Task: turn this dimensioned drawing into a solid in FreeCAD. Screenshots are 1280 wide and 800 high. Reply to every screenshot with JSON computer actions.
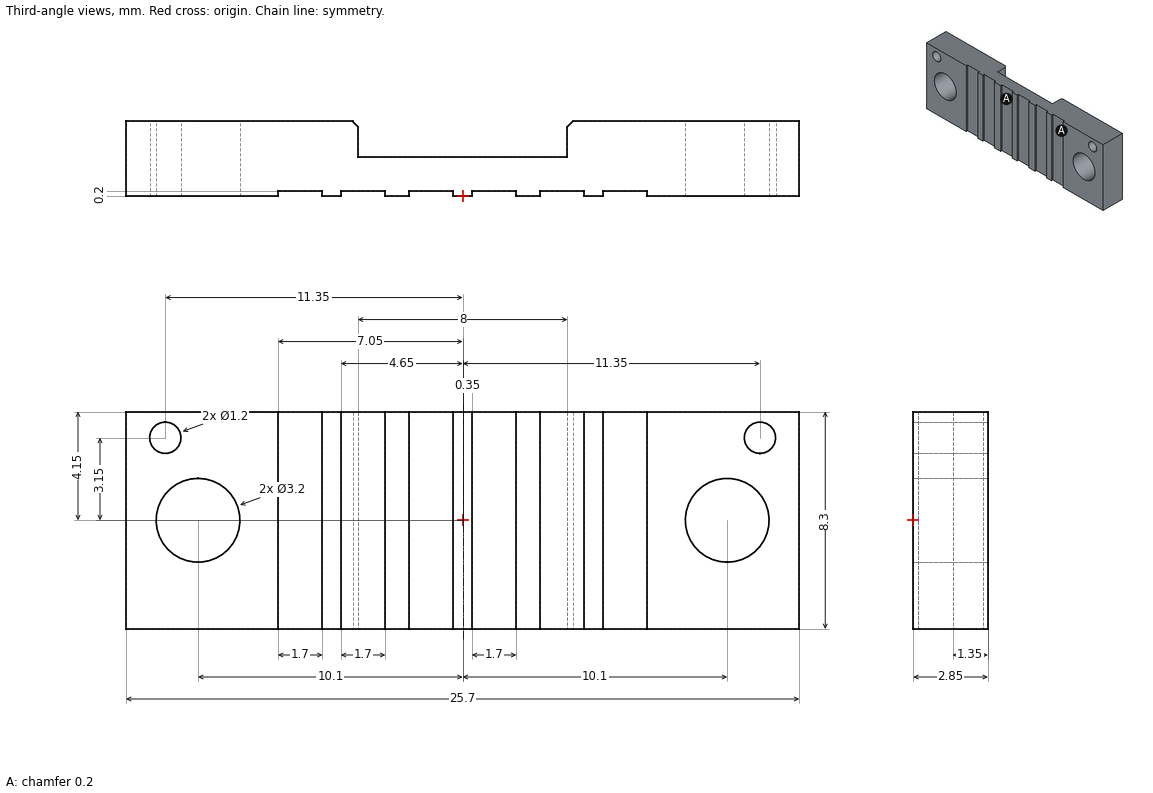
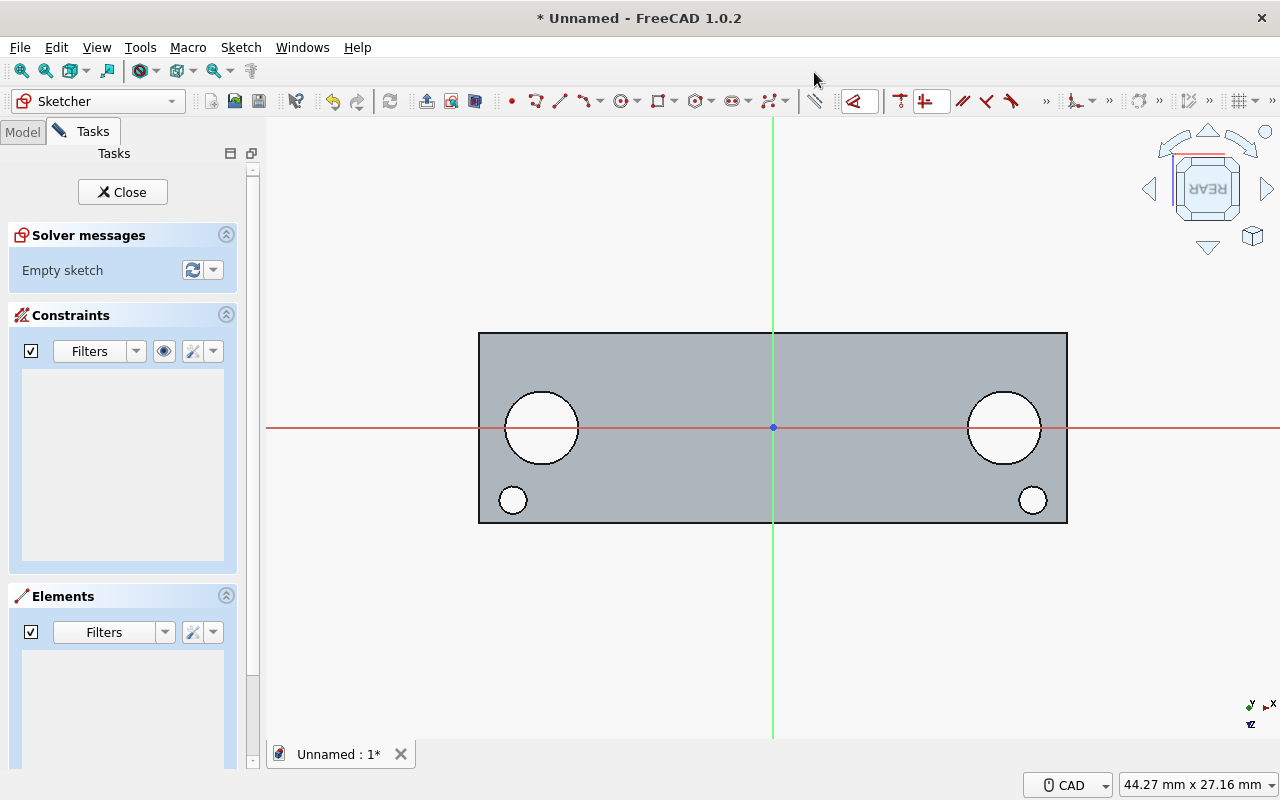
{"action": "scroll", "coordinate": [829, 428], "scroll_direction": "up", "scroll_amount": 4}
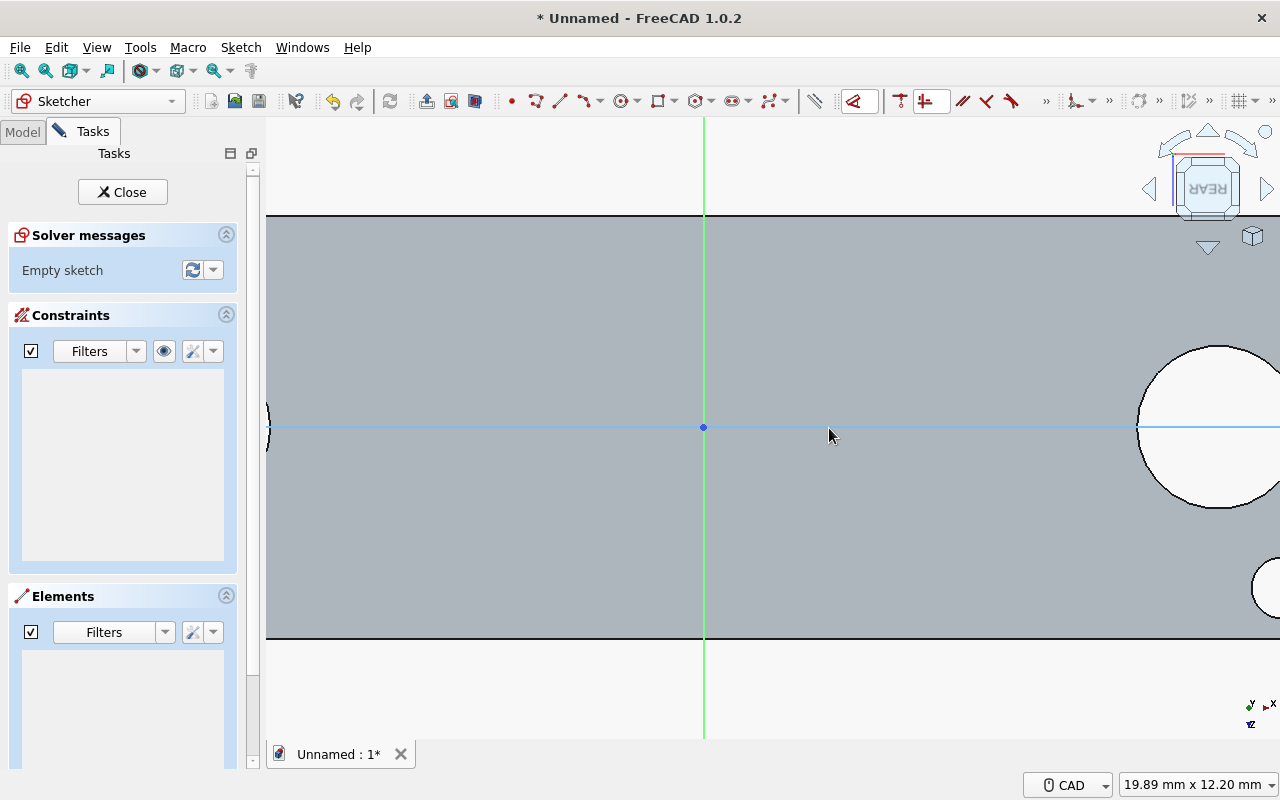
{"action": "key", "text": "g v"}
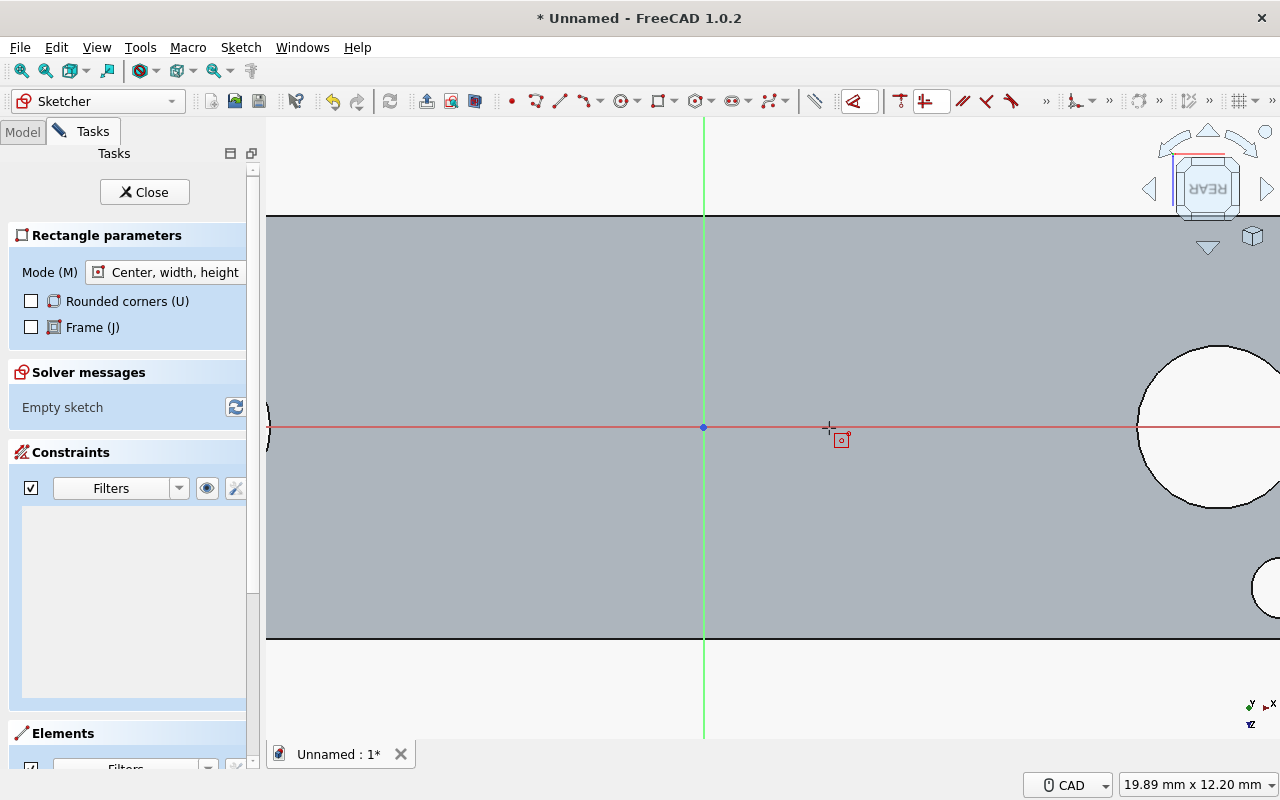
{"action": "left_click", "coordinate": [704, 427]}
{"action": "left_click", "coordinate": [908, 216]}
{"action": "key", "text": "Escape"}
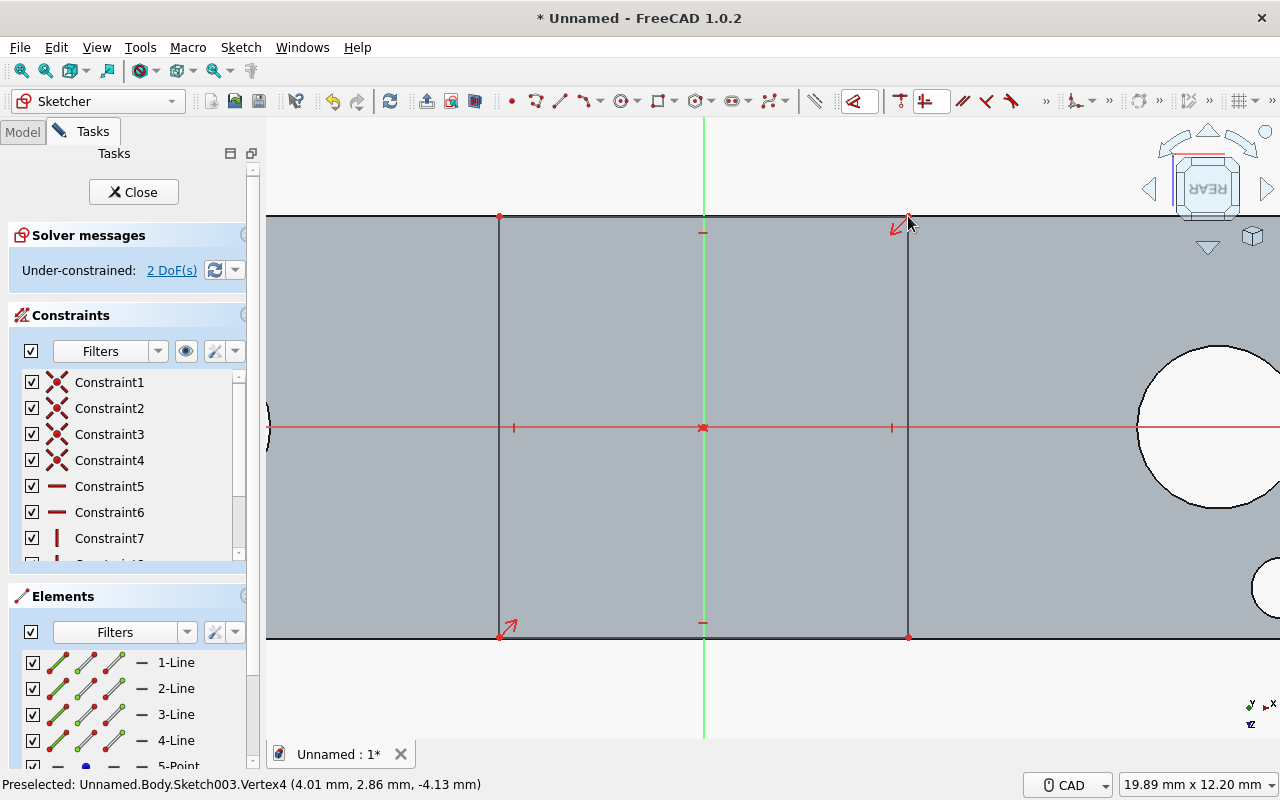
{"action": "key", "text": "d"}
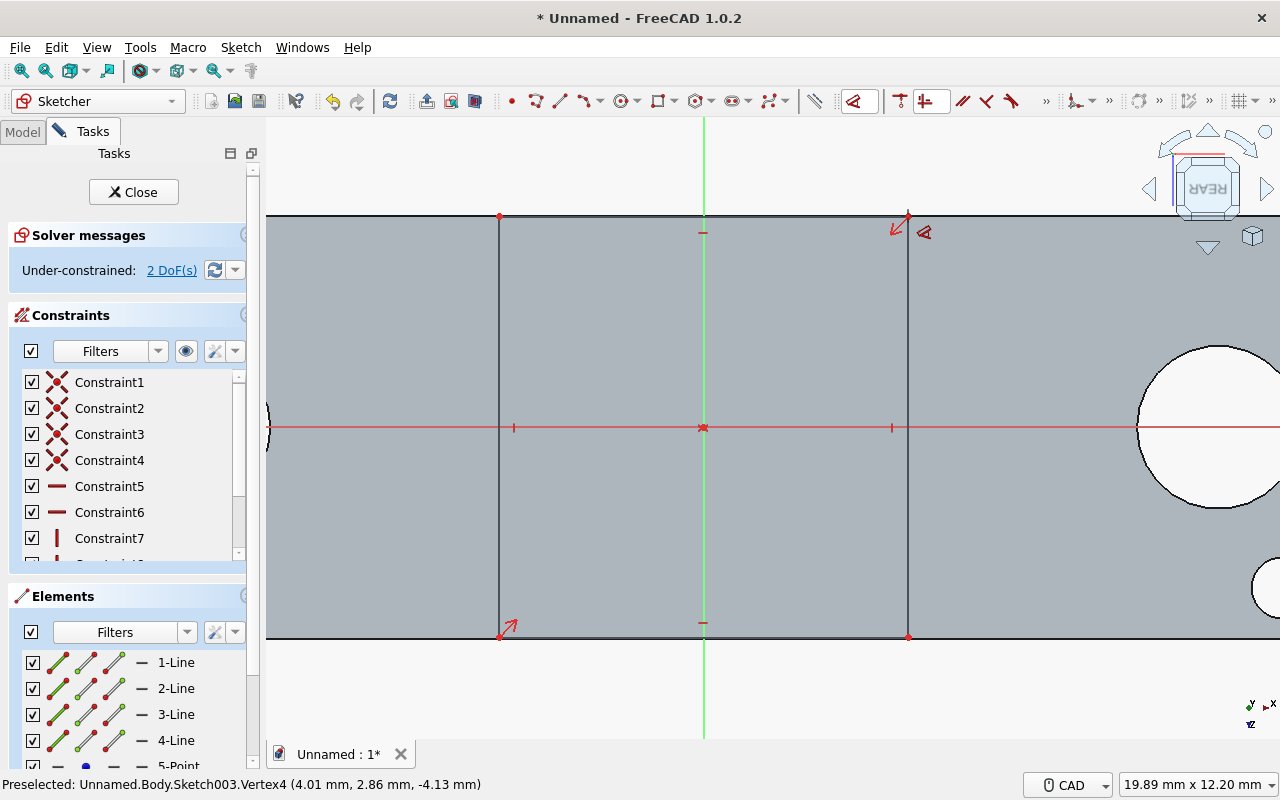
{"action": "left_click", "coordinate": [622, 638]}
{"action": "left_click", "coordinate": [610, 672]}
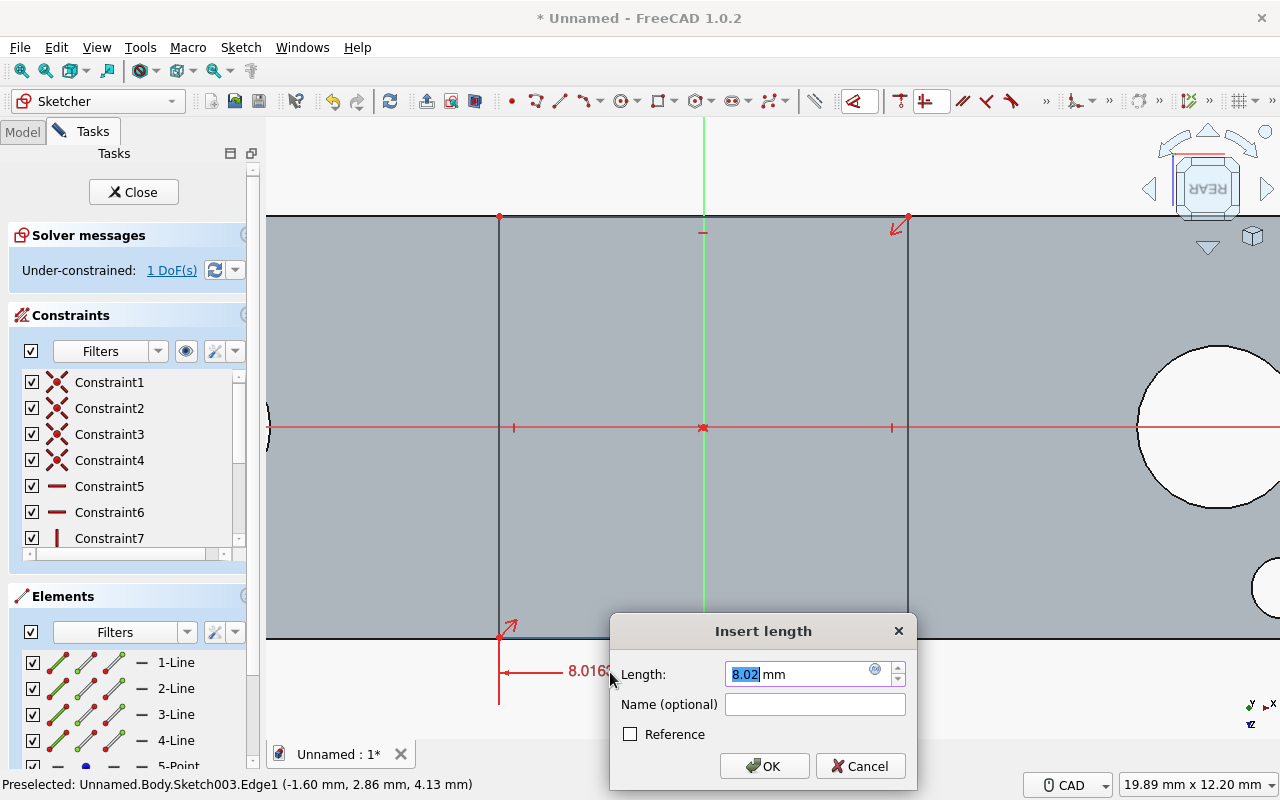
{"action": "type", "text": "8"}
{"action": "key", "text": "Return"}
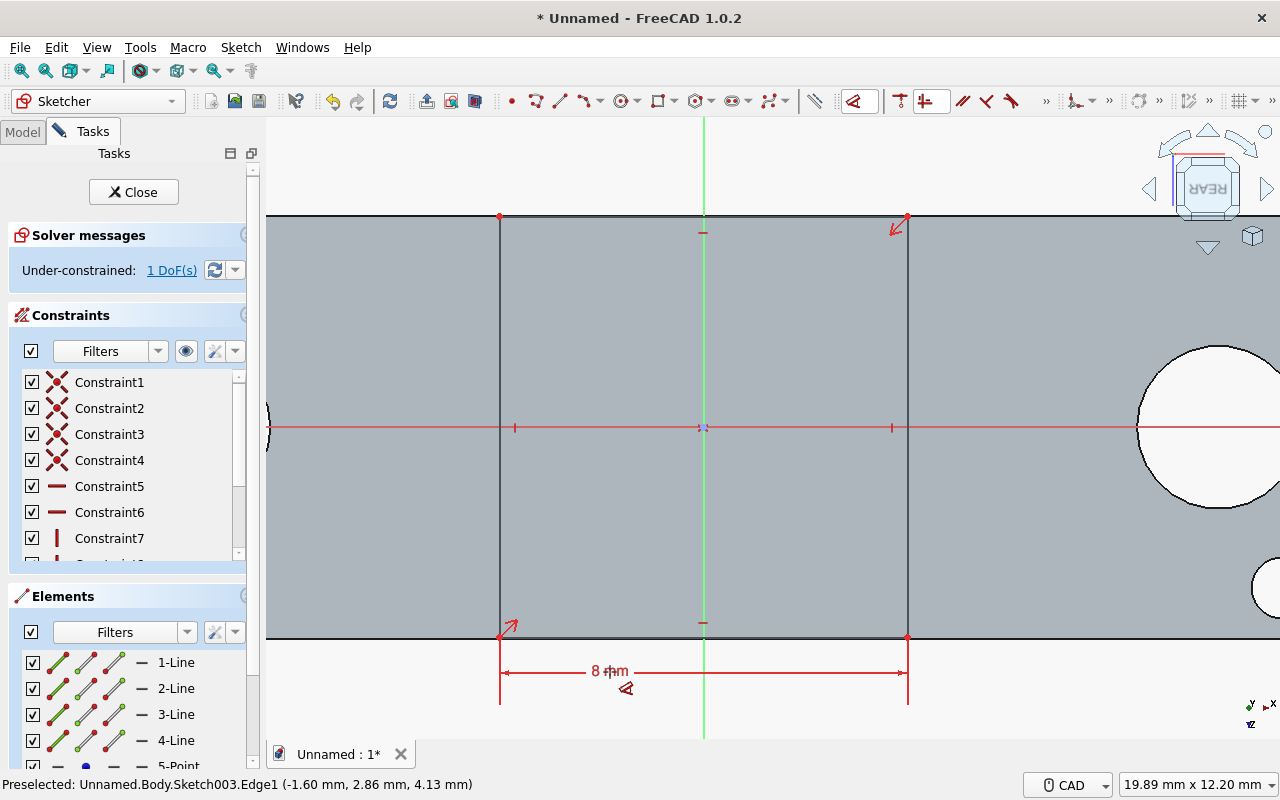
{"action": "left_click", "coordinate": [908, 512]}
{"action": "left_click", "coordinate": [942, 331]}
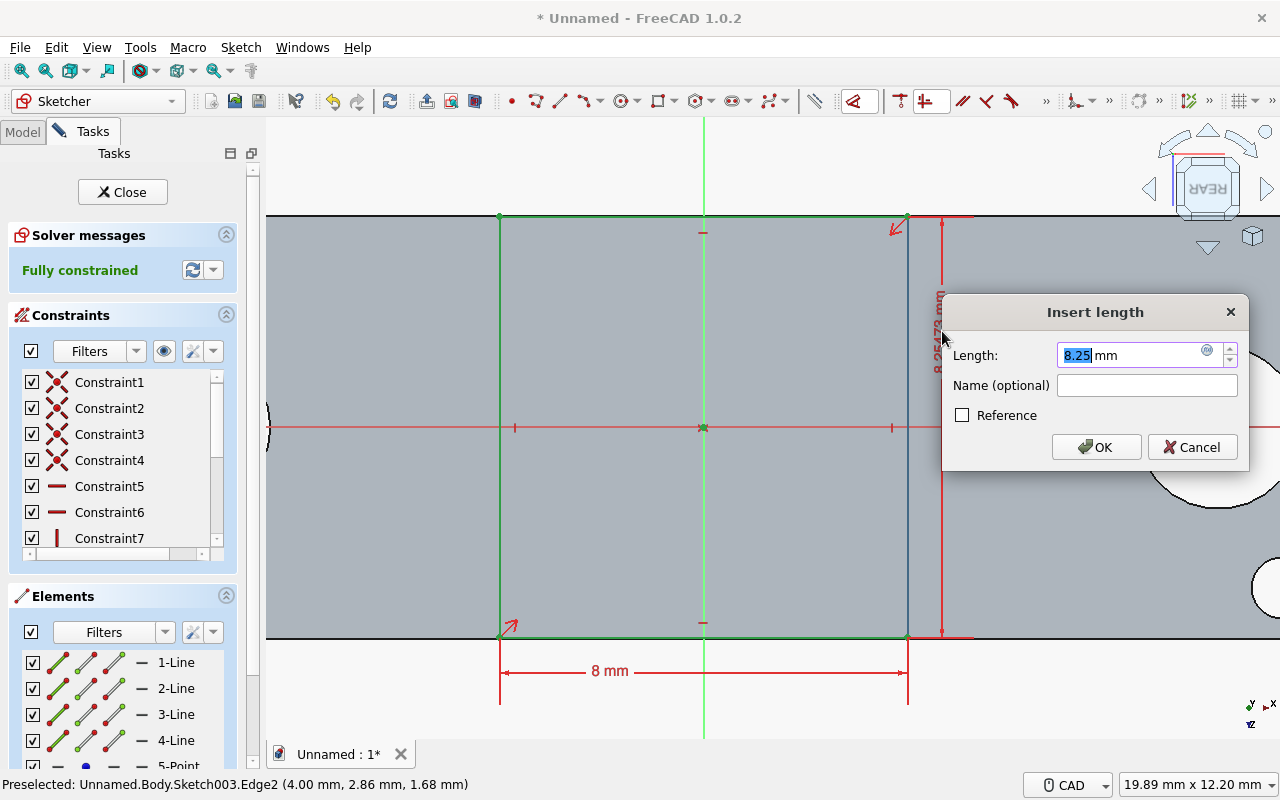
{"action": "type", "text": "8.3"}
{"action": "key", "text": "Return"}
{"action": "key", "text": "Escape"}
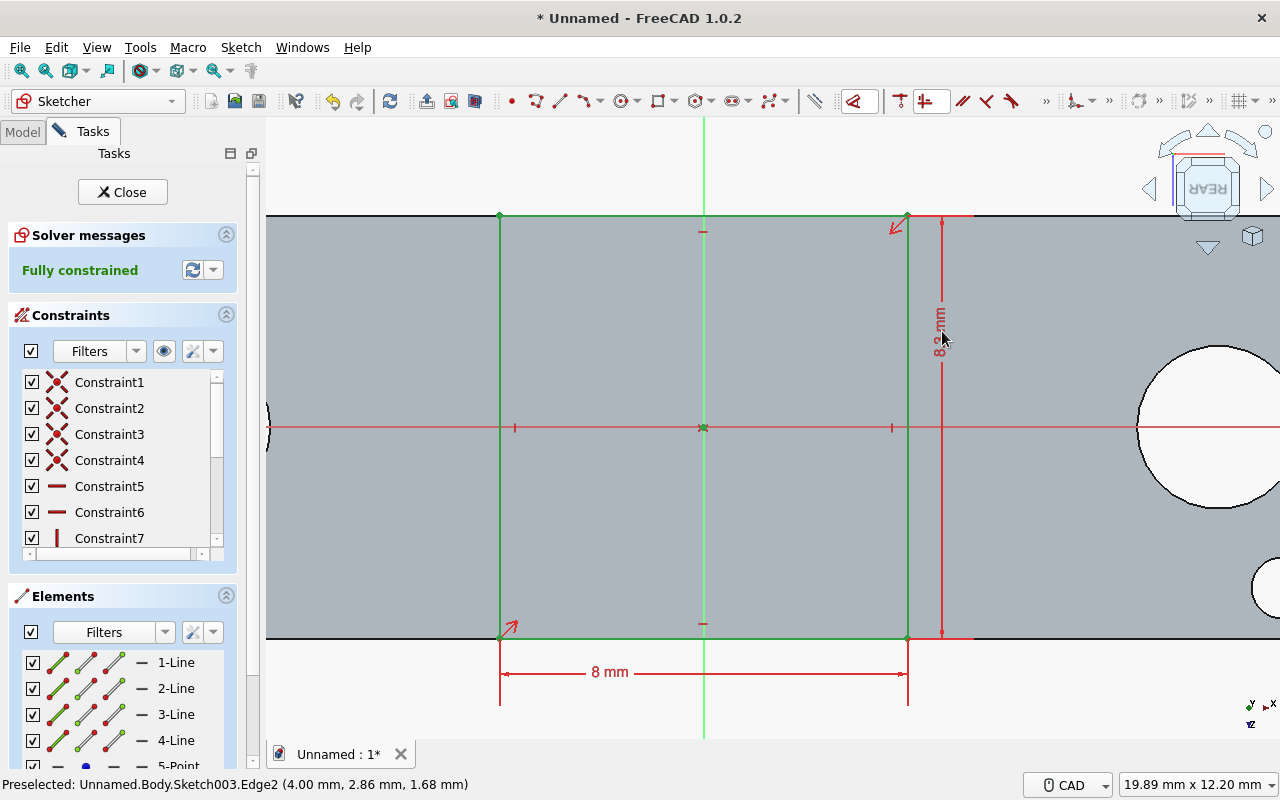
{"action": "left_click", "coordinate": [123, 192]}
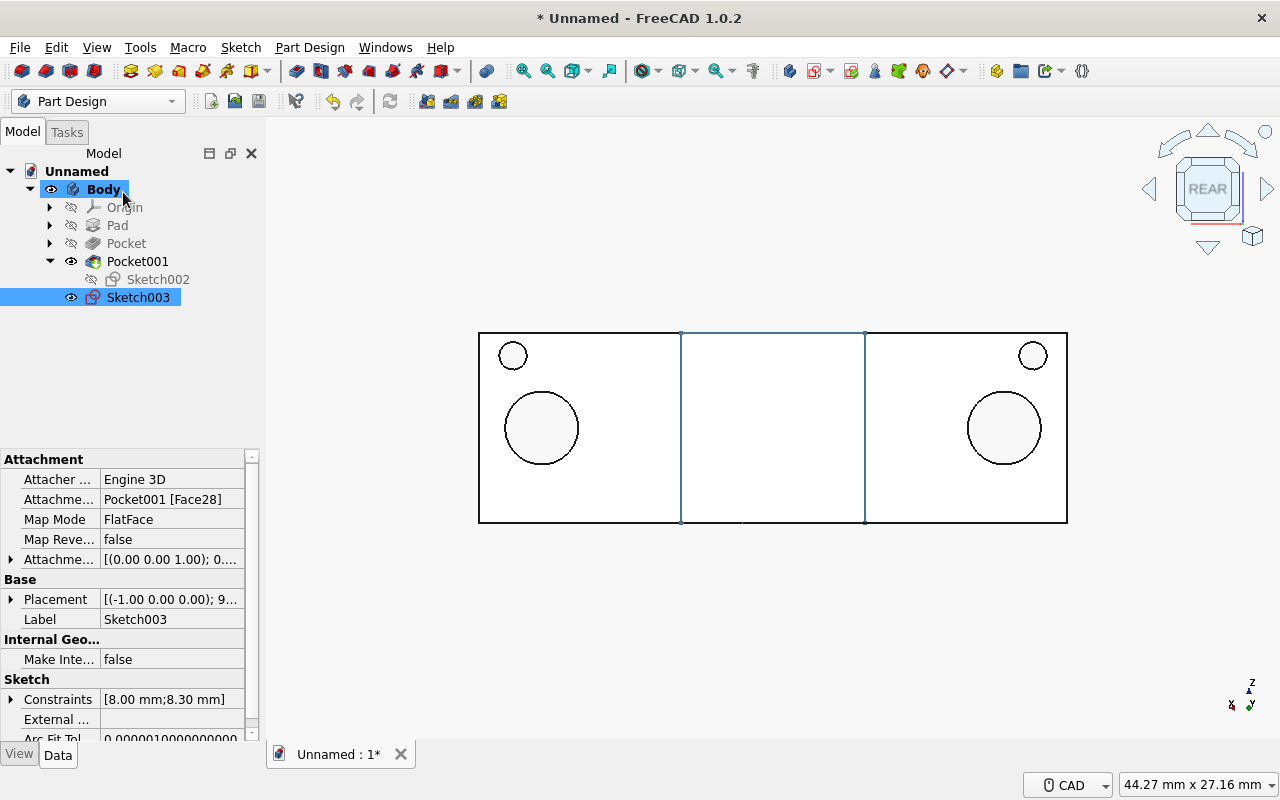
{"action": "left_click", "coordinate": [298, 72]}